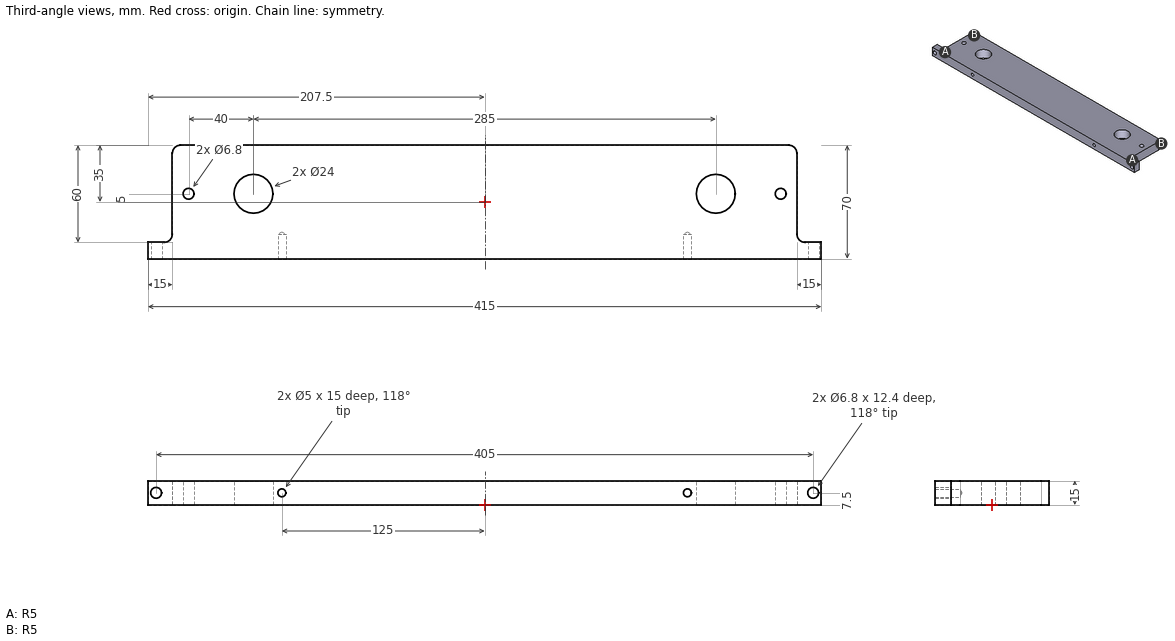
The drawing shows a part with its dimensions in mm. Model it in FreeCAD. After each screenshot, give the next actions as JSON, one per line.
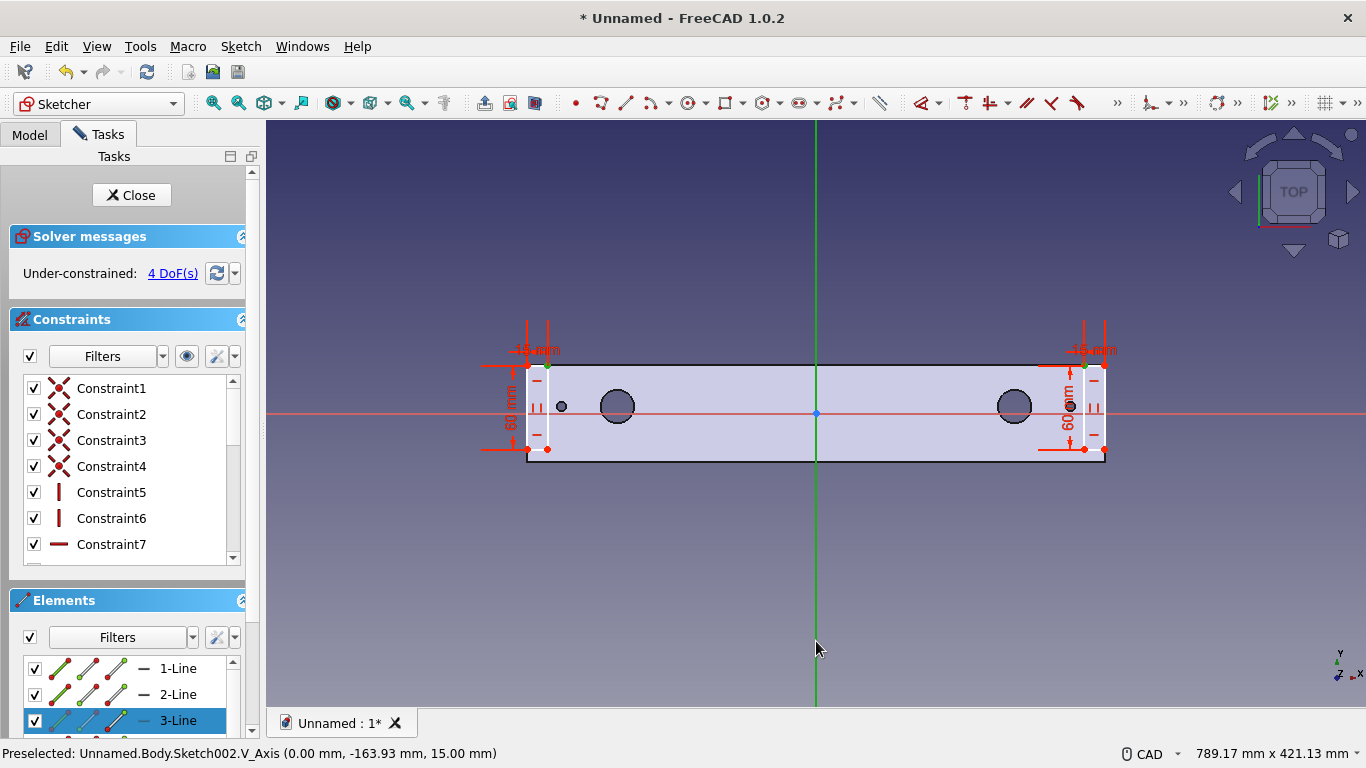
{"action": "key", "text": "s"}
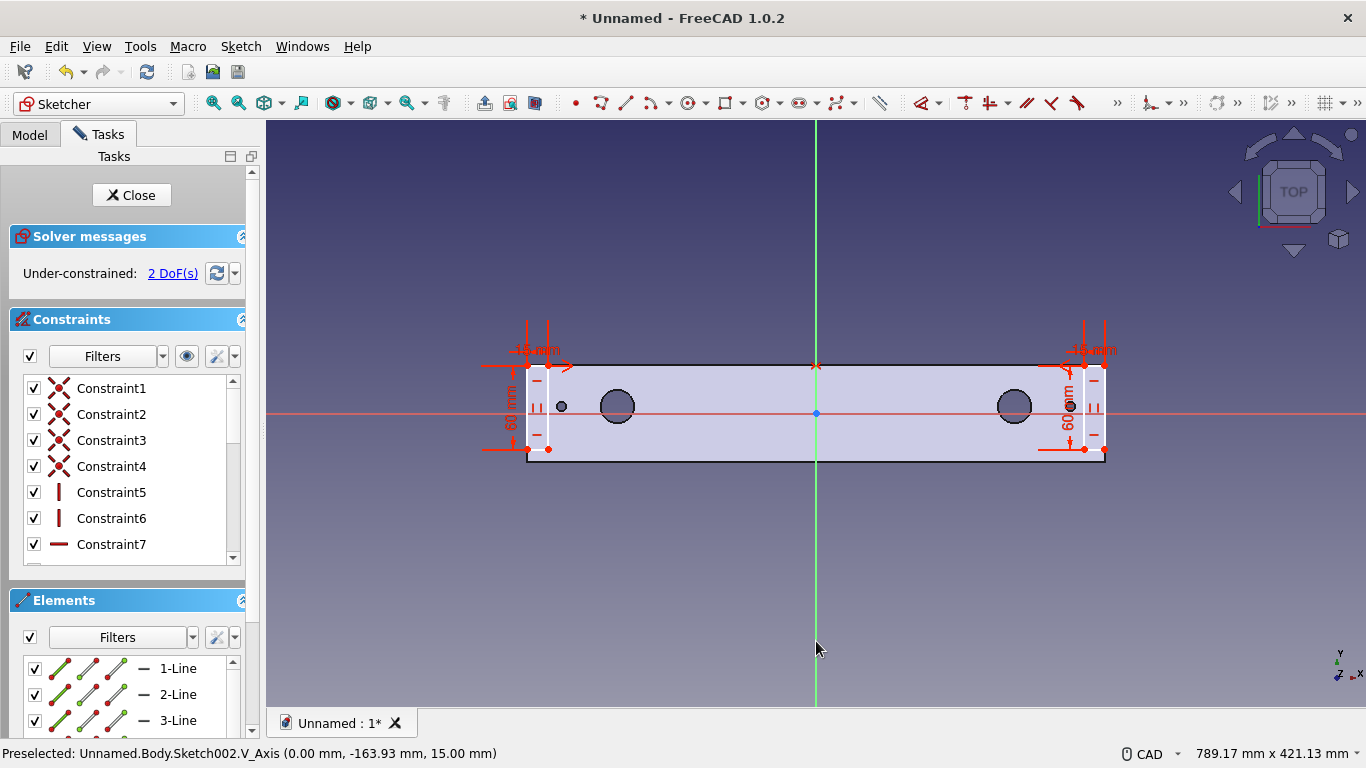
{"action": "key", "text": "d"}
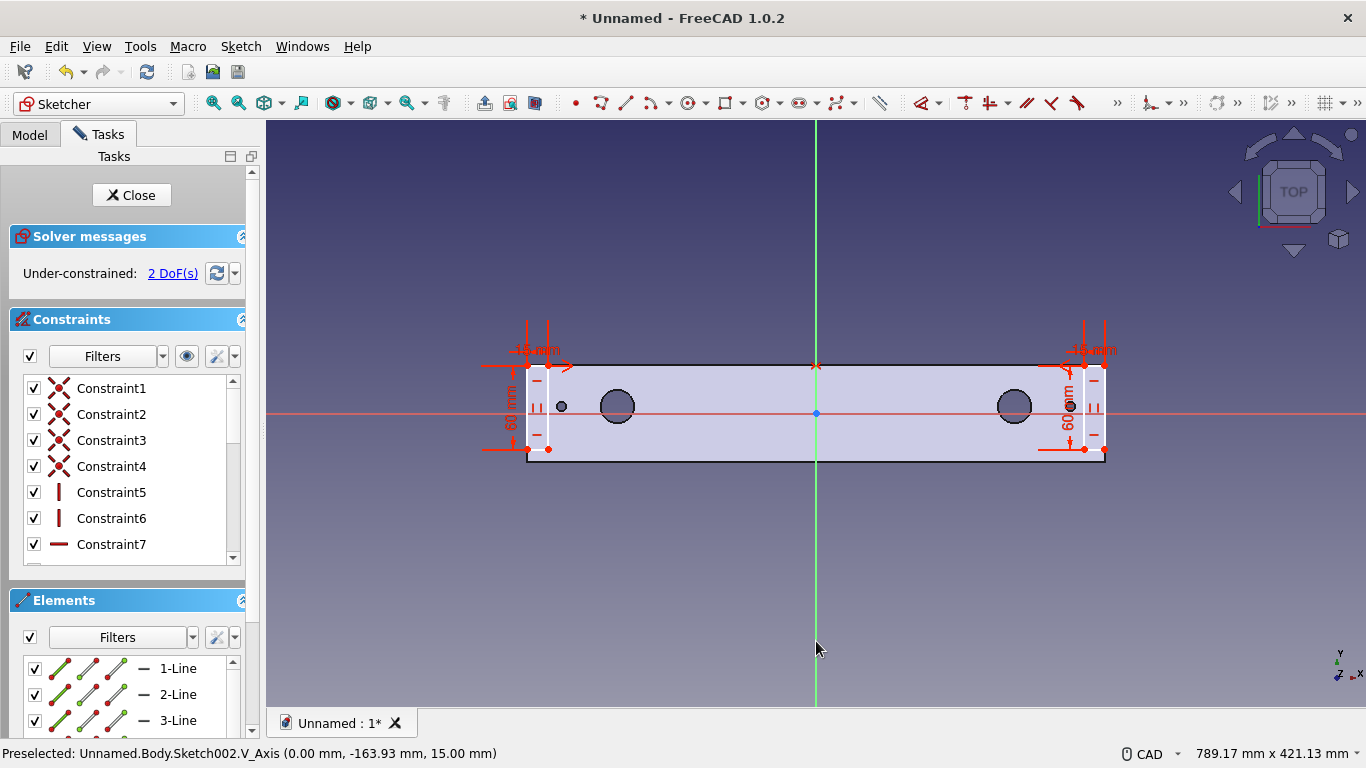
{"action": "left_click", "coordinate": [527, 366]}
{"action": "left_click", "coordinate": [493, 390]}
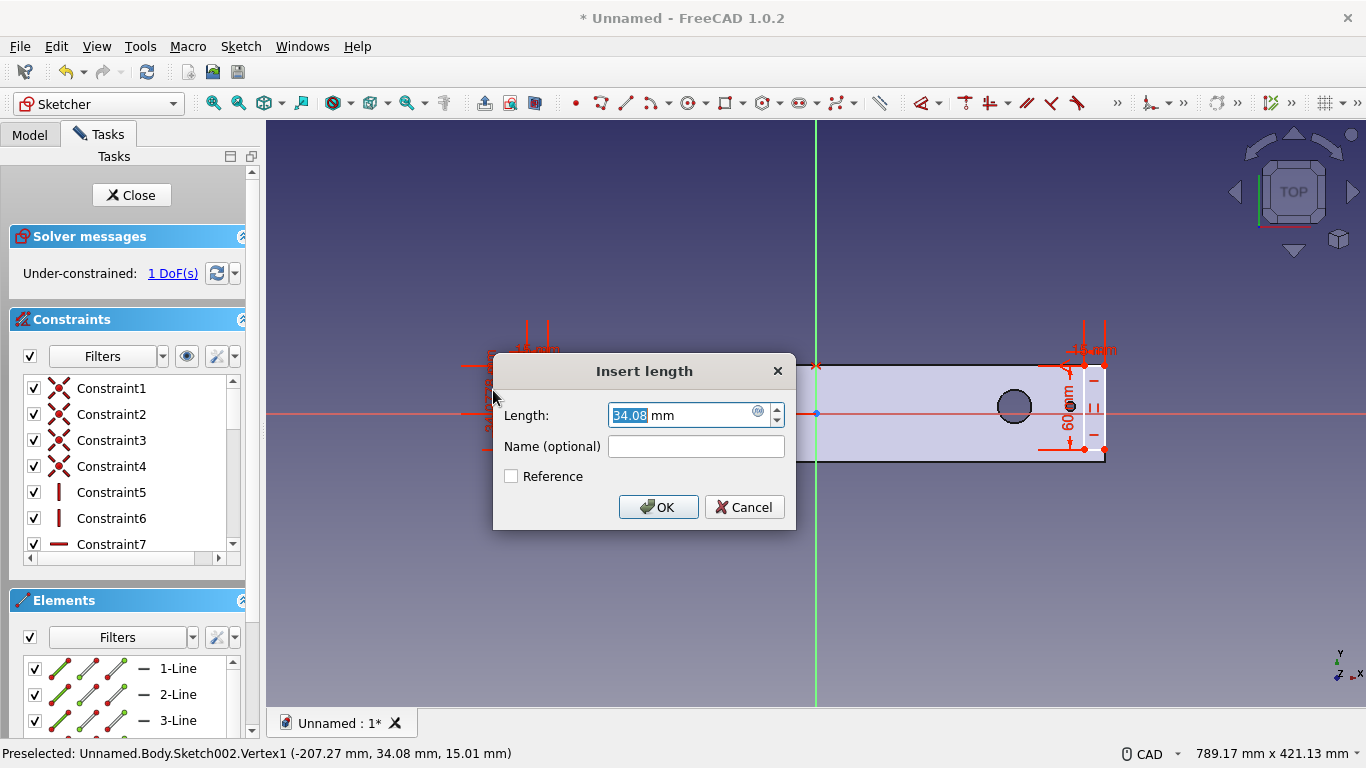
{"action": "type", "text": "35"}
{"action": "key", "text": "Return"}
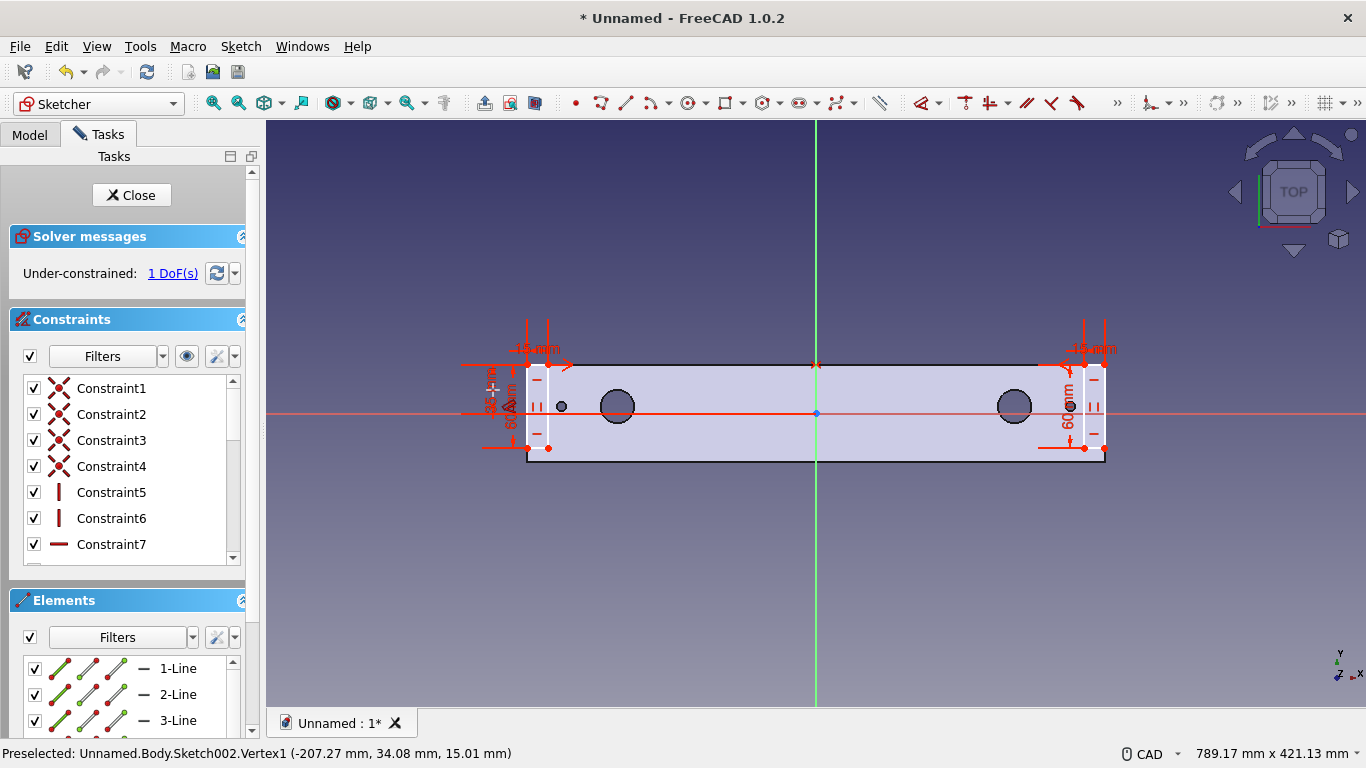
{"action": "left_click", "coordinate": [527, 365]}
{"action": "left_click", "coordinate": [672, 331]}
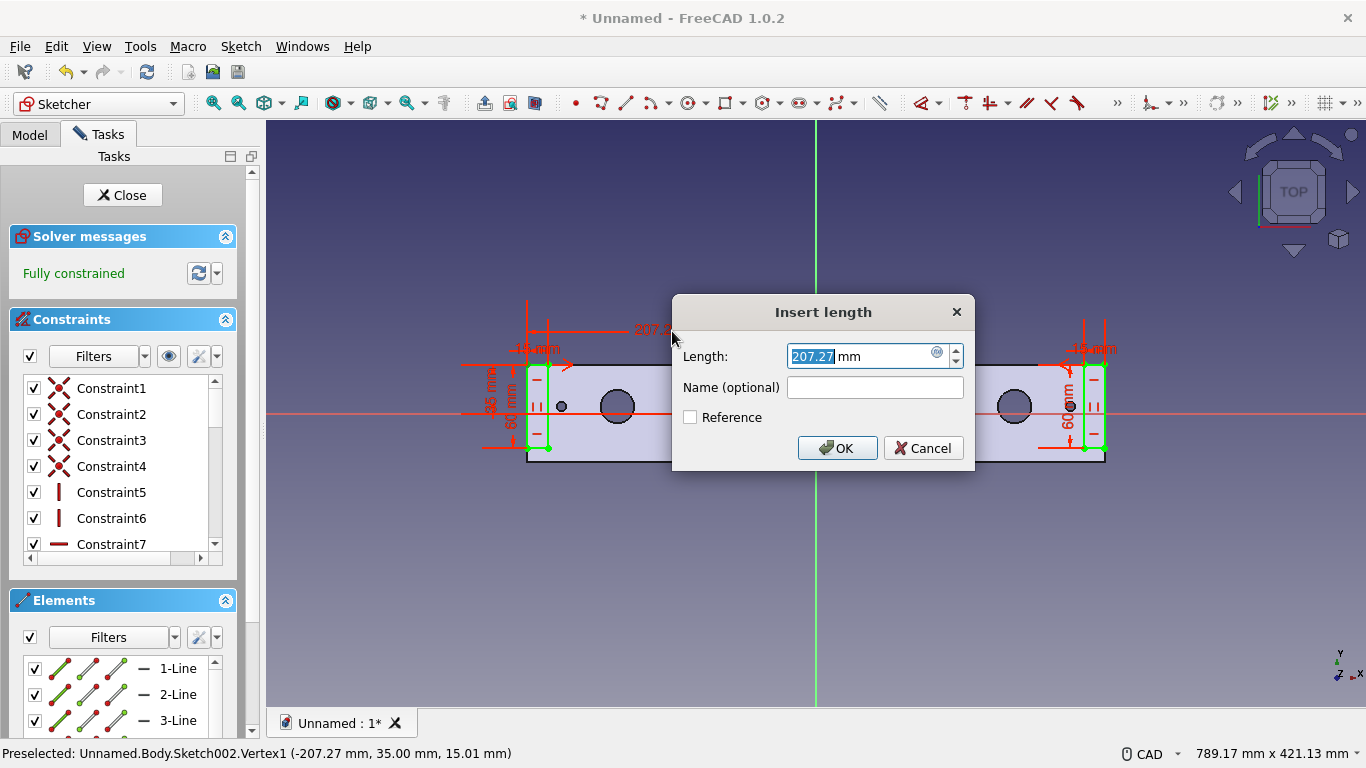
{"action": "type", "text": "207.5"}
{"action": "key", "text": "Return"}
{"action": "key", "text": "Escape"}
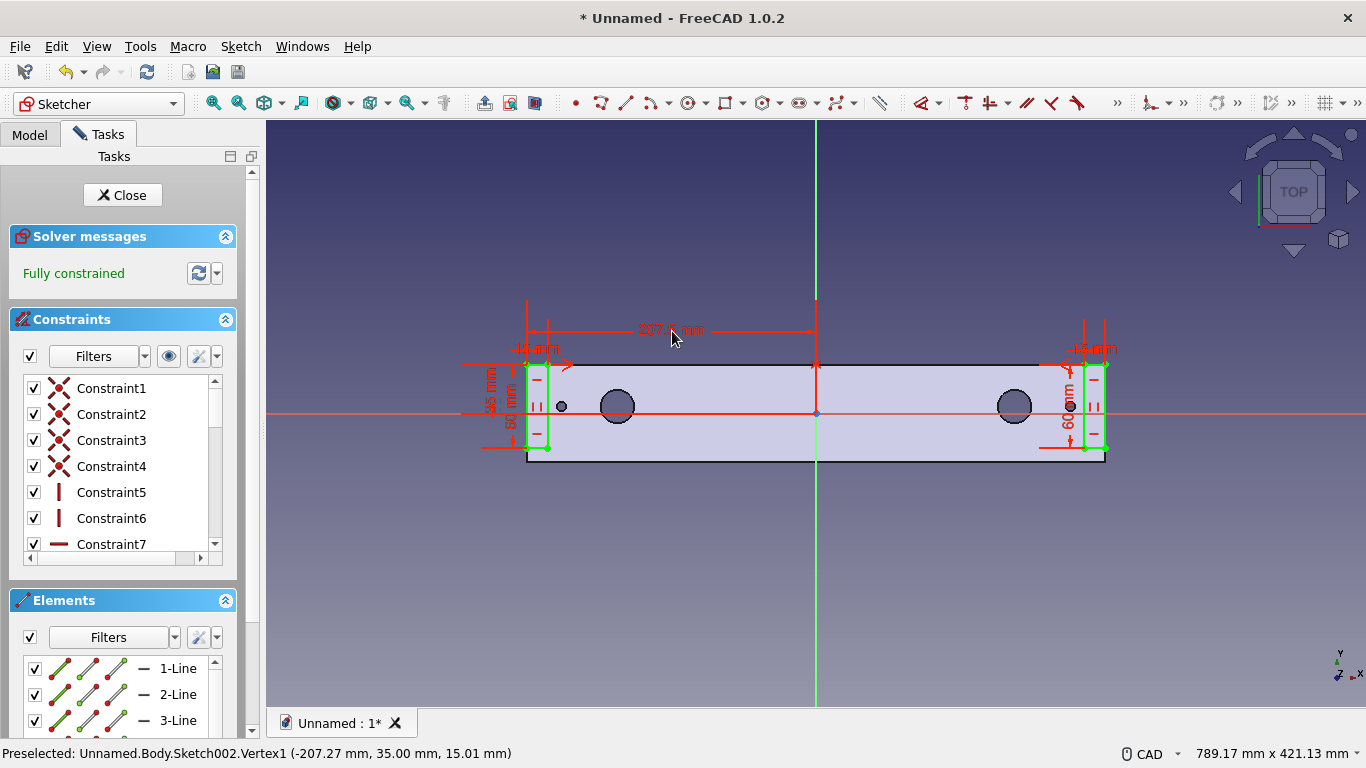
{"action": "left_click", "coordinate": [123, 195]}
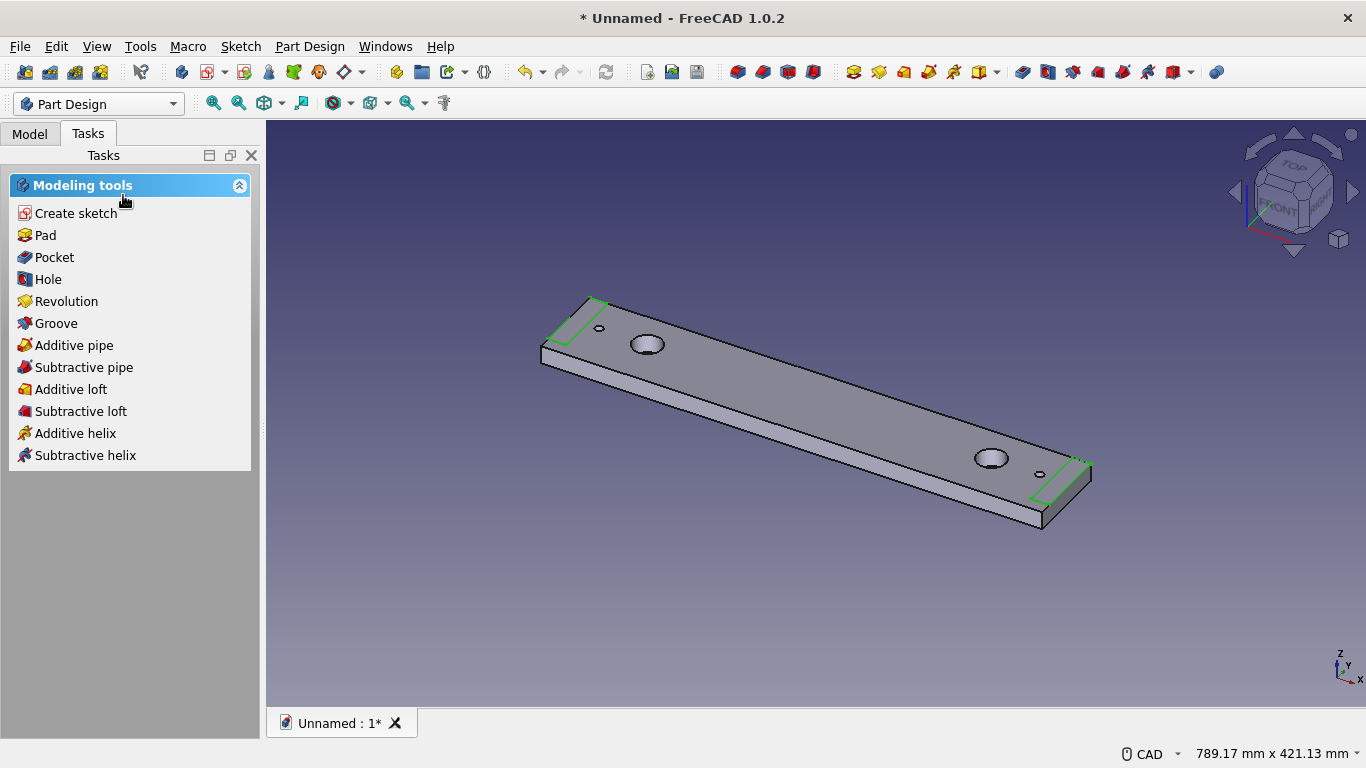
{"action": "left_click", "coordinate": [1023, 72]}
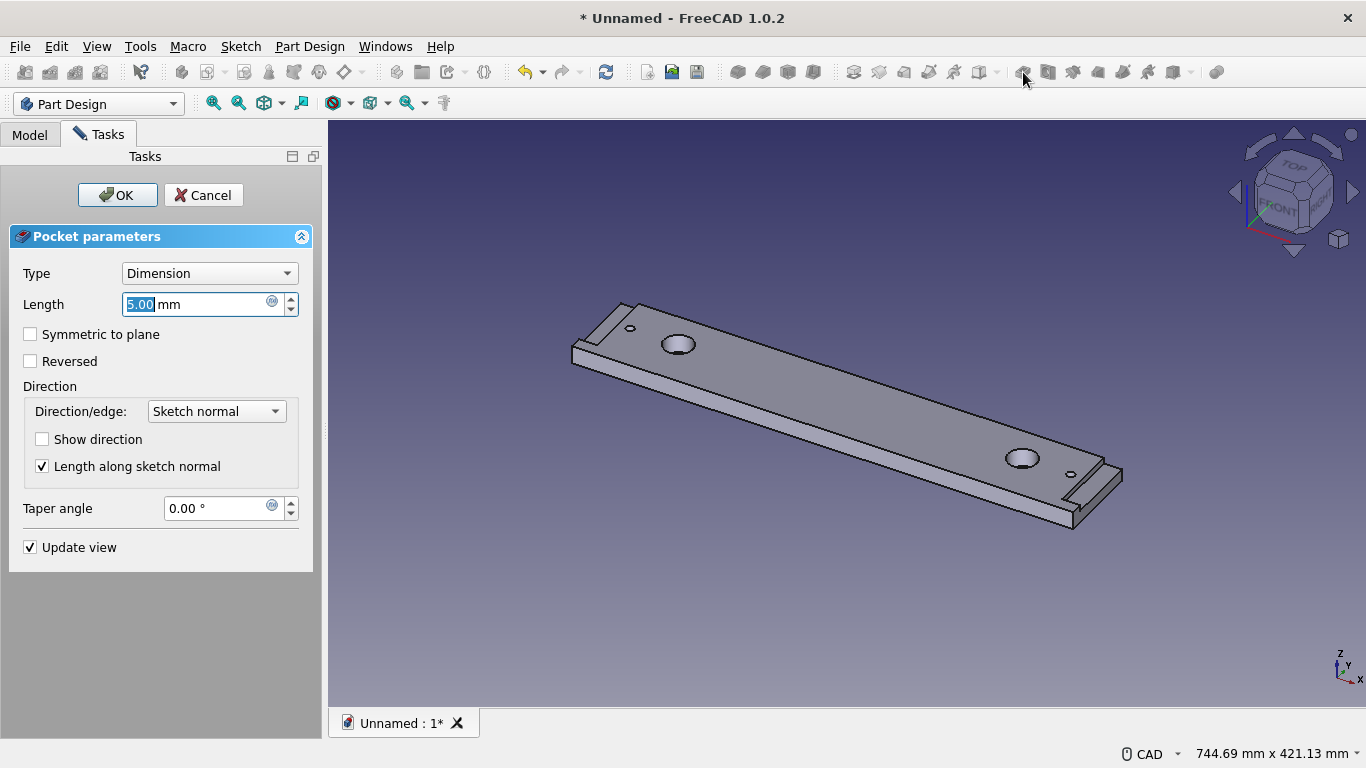
{"action": "left_click", "coordinate": [210, 274]}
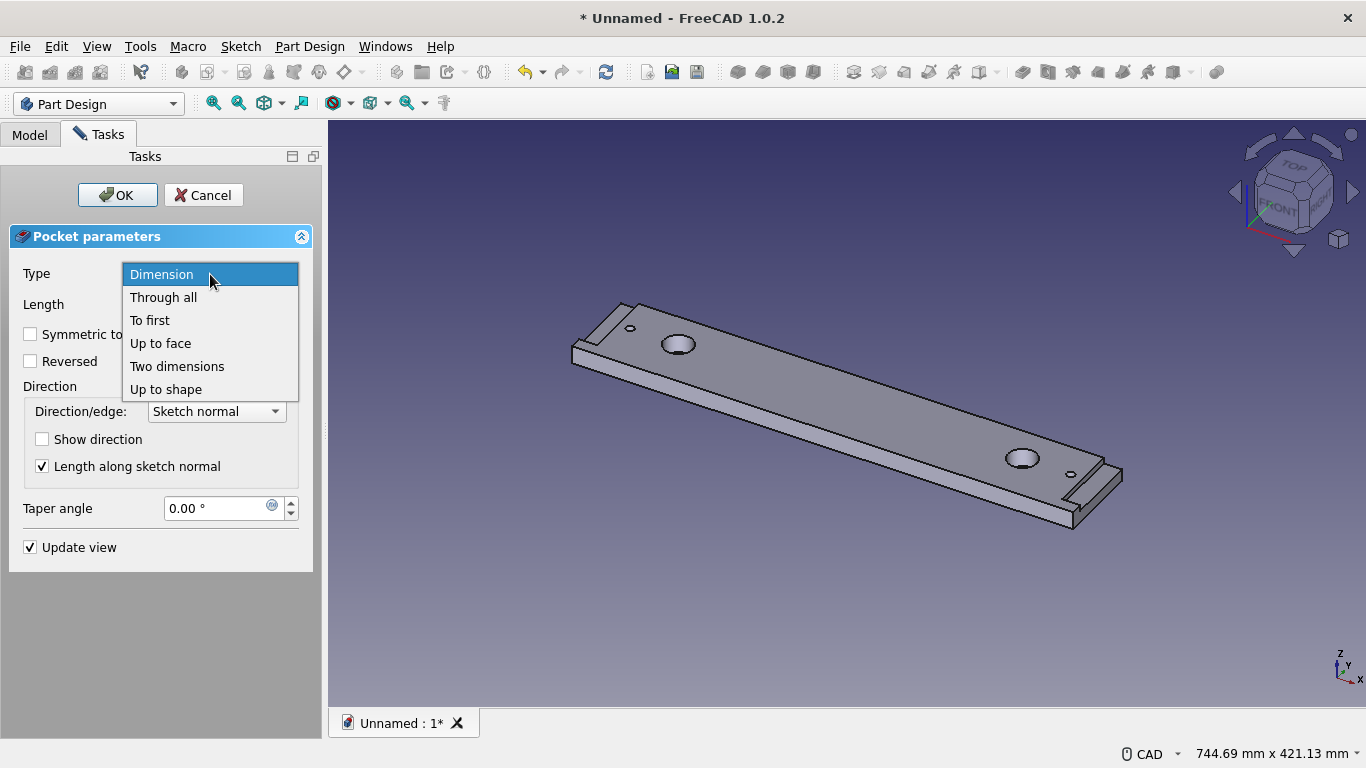
{"action": "left_click", "coordinate": [208, 298]}